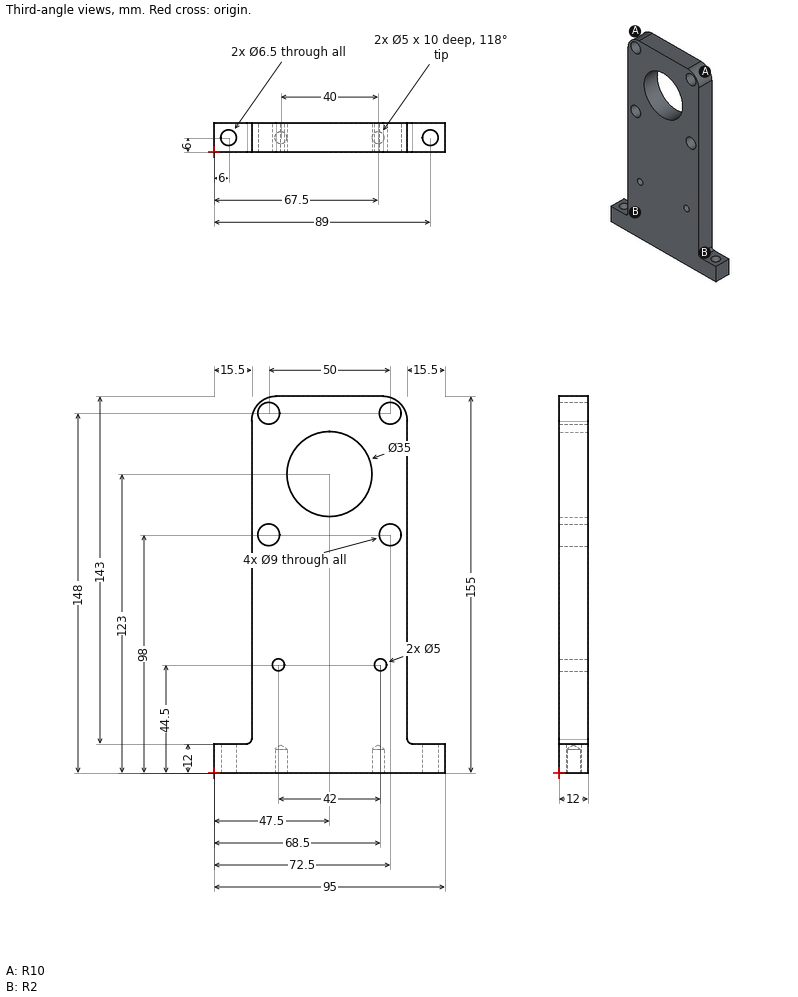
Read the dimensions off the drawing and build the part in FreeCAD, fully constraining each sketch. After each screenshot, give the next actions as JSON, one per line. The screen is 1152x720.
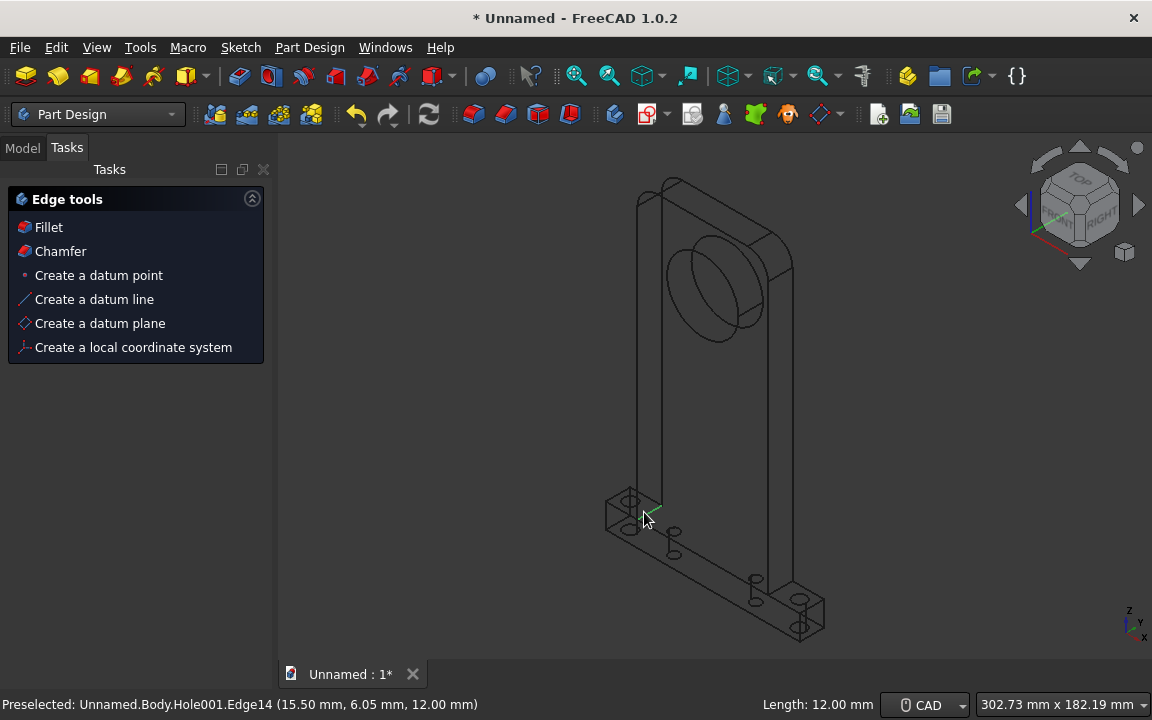
{"action": "left_click", "coordinate": [780, 587], "text": "ctrl"}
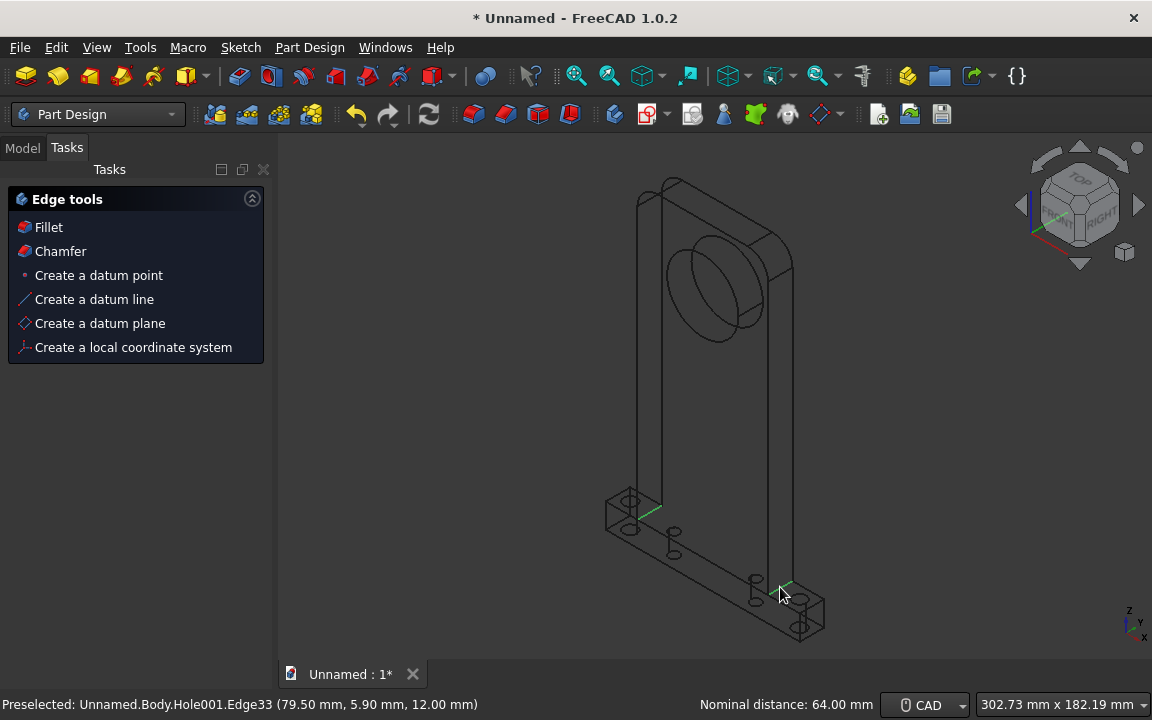
{"action": "key", "text": "v 1"}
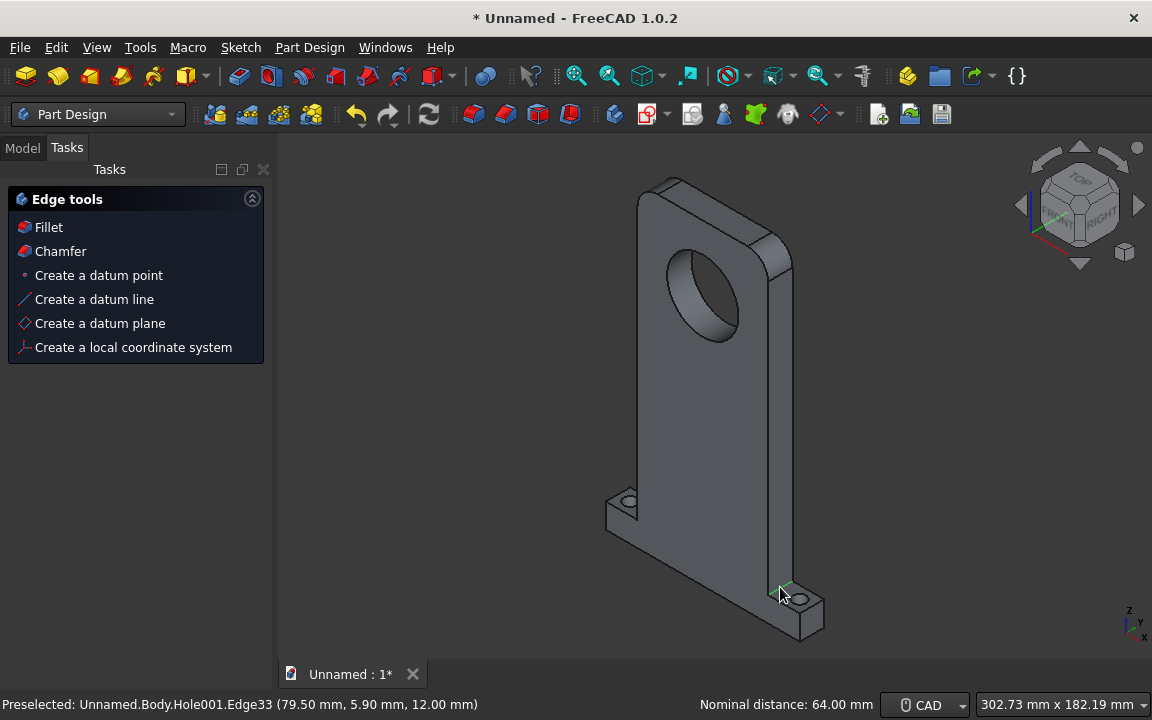
{"action": "left_click", "coordinate": [474, 114]}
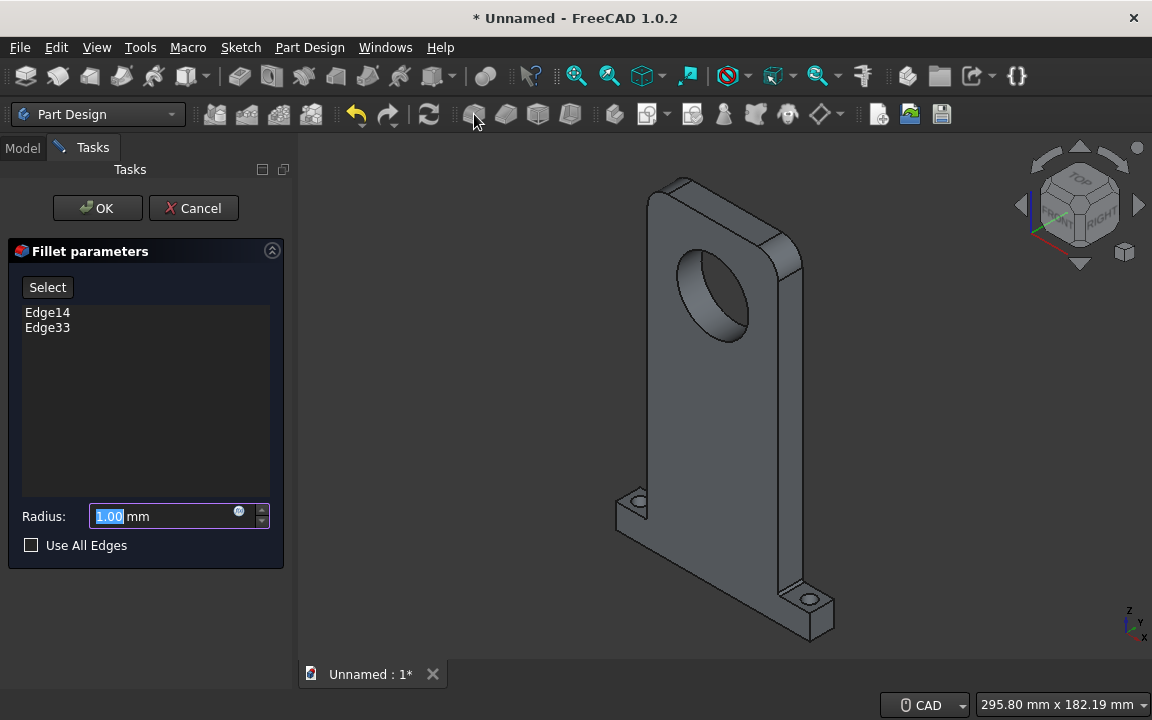
{"action": "type", "text": "2"}
{"action": "key", "text": "Tab"}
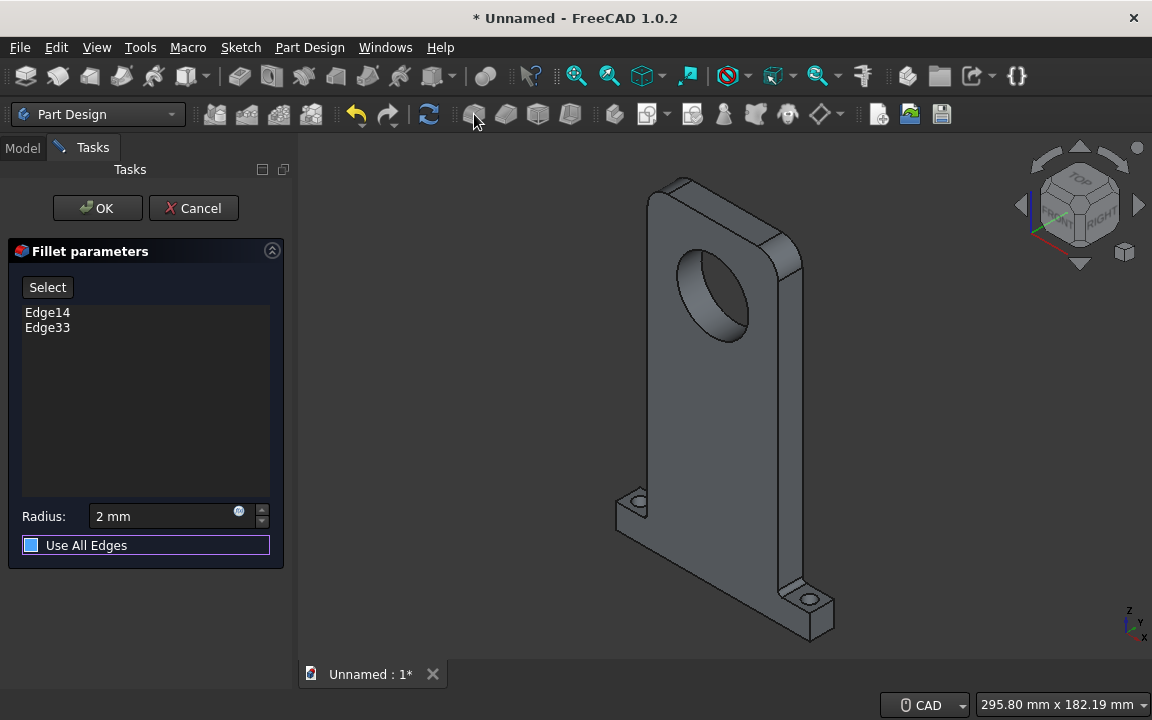
{"action": "left_click", "coordinate": [98, 208]}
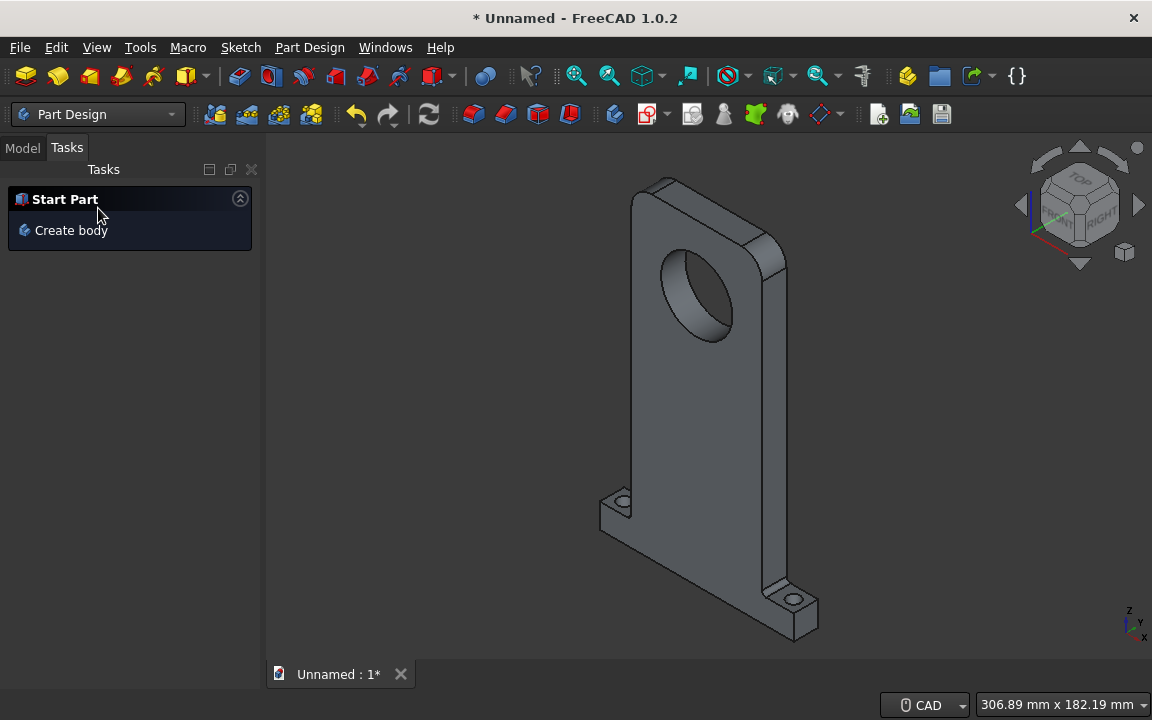
{"action": "left_click", "coordinate": [648, 114]}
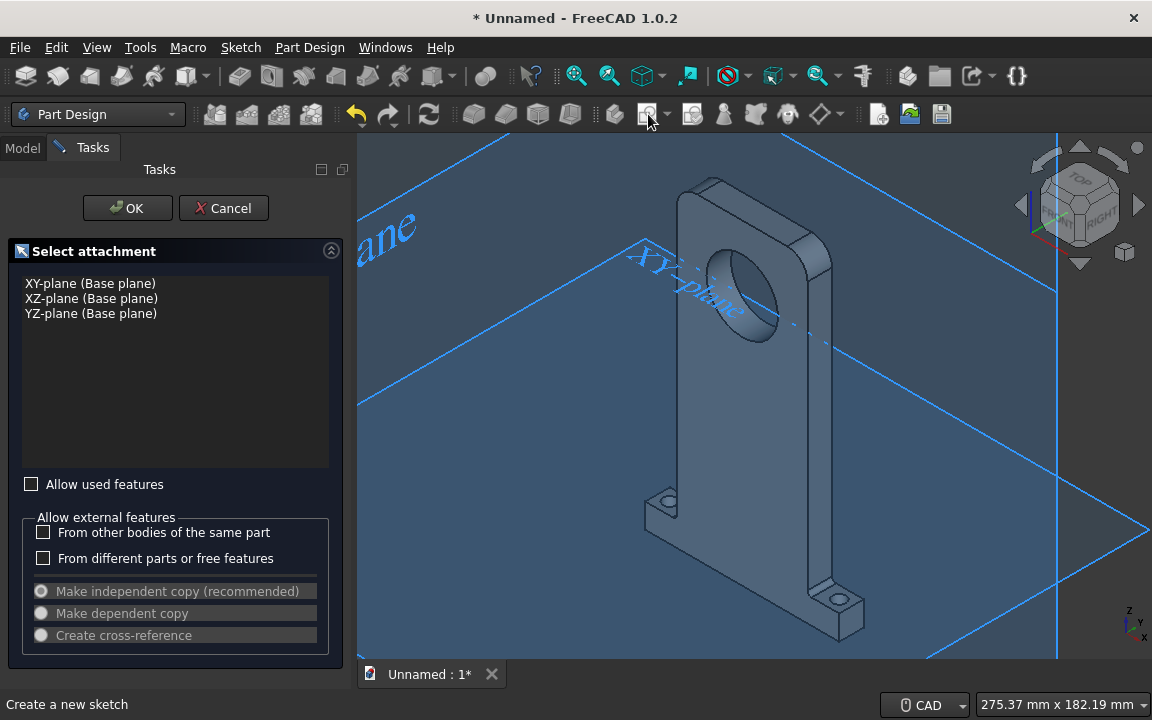
{"action": "left_click", "coordinate": [82, 298]}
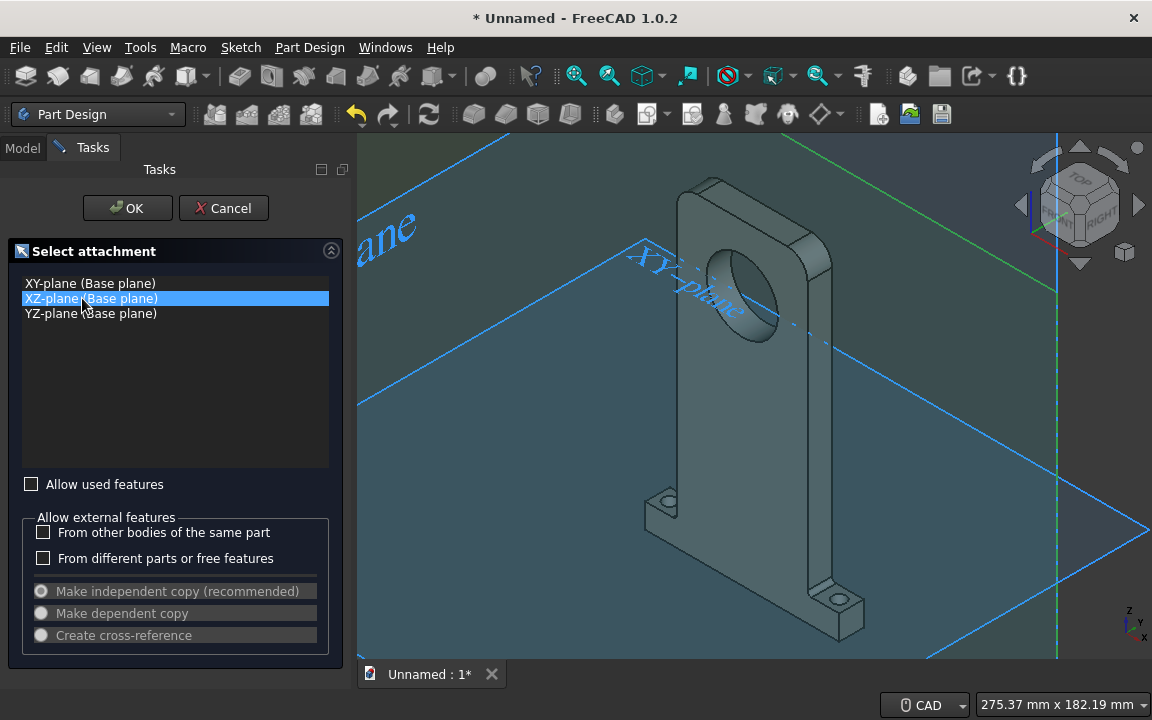
{"action": "left_click", "coordinate": [128, 208]}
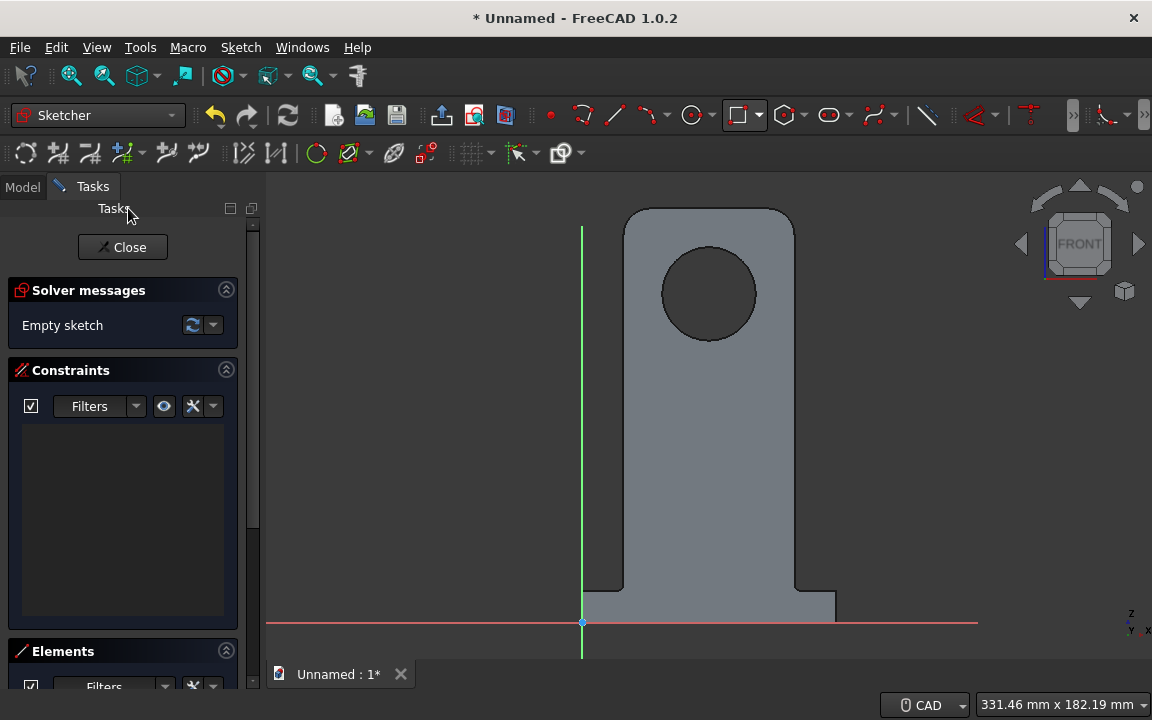
{"action": "scroll", "coordinate": [640, 416], "scroll_direction": "down", "scroll_amount": 5}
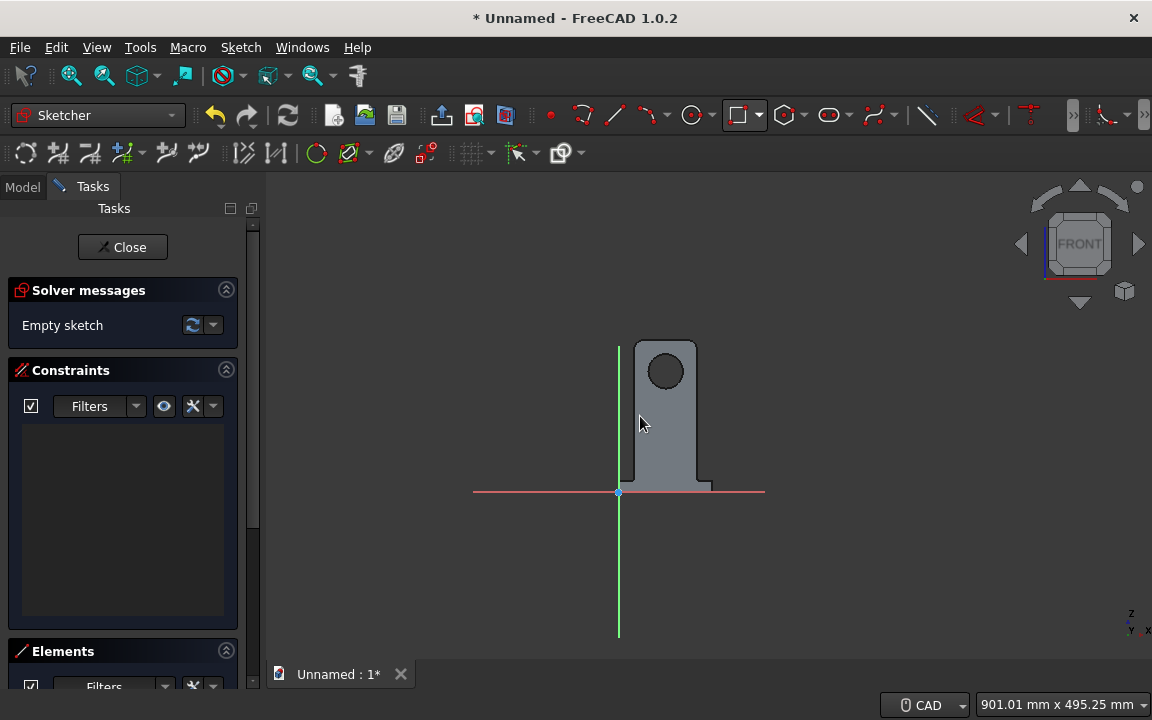
{"action": "scroll", "coordinate": [656, 480], "scroll_direction": "up", "scroll_amount": 9}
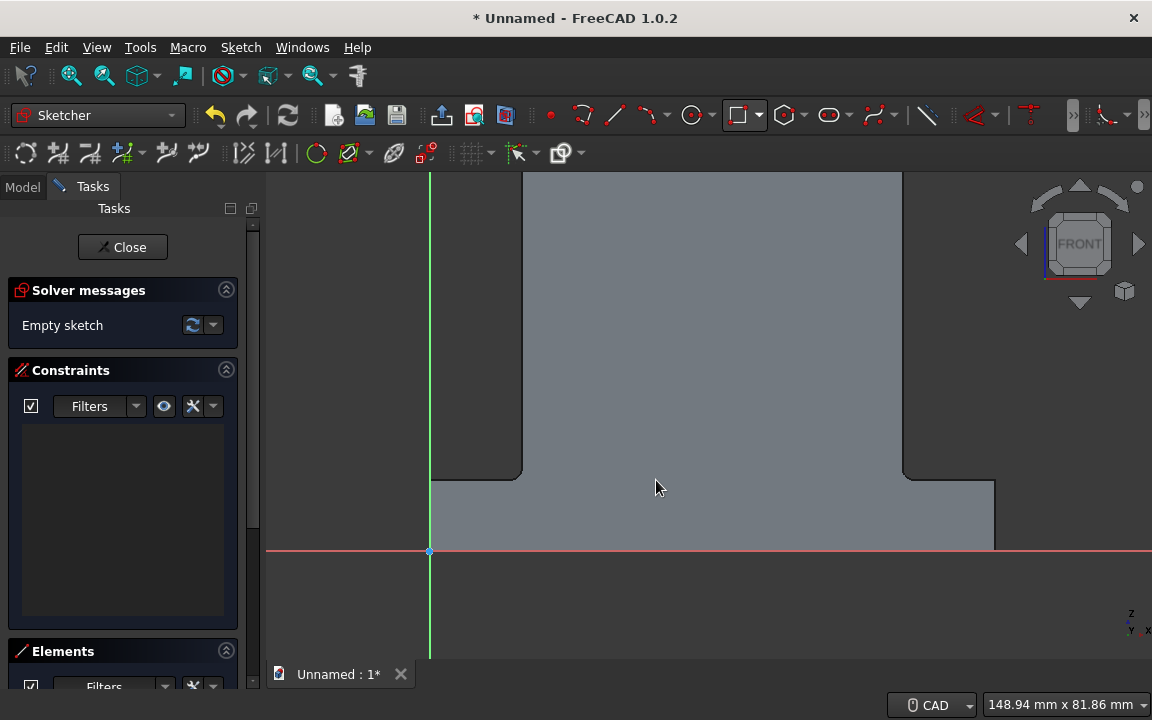
{"action": "left_click", "coordinate": [692, 116]}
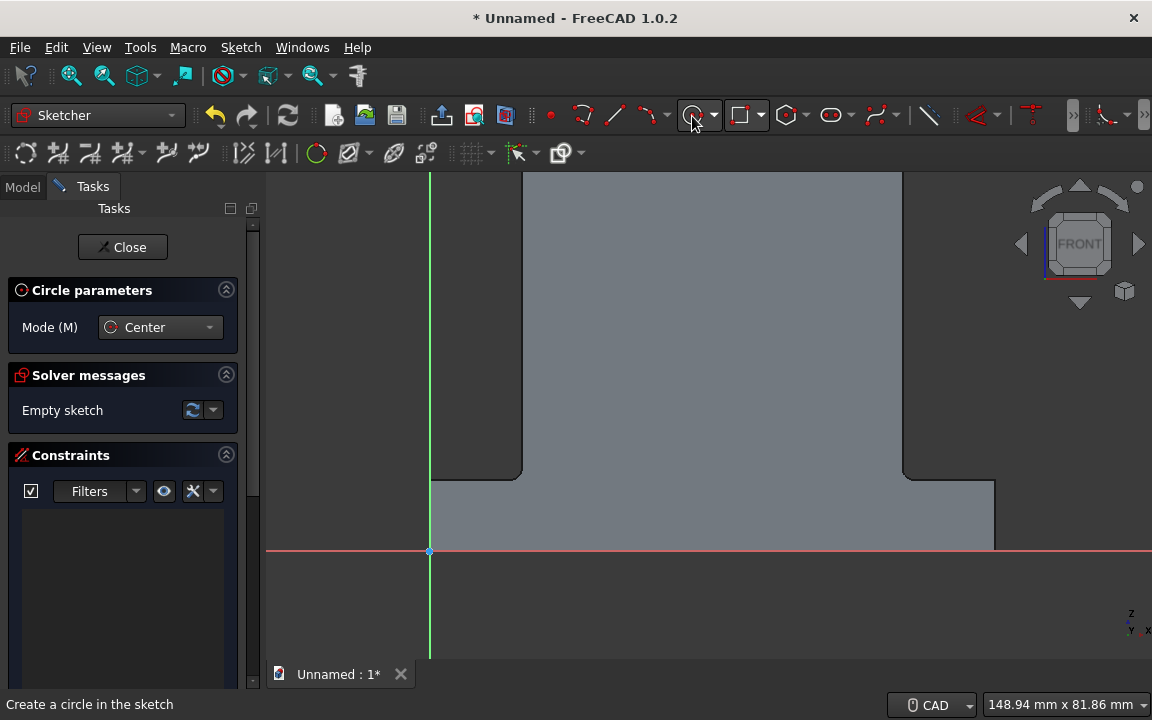
{"action": "scroll", "coordinate": [837, 287], "scroll_direction": "up", "scroll_amount": 3}